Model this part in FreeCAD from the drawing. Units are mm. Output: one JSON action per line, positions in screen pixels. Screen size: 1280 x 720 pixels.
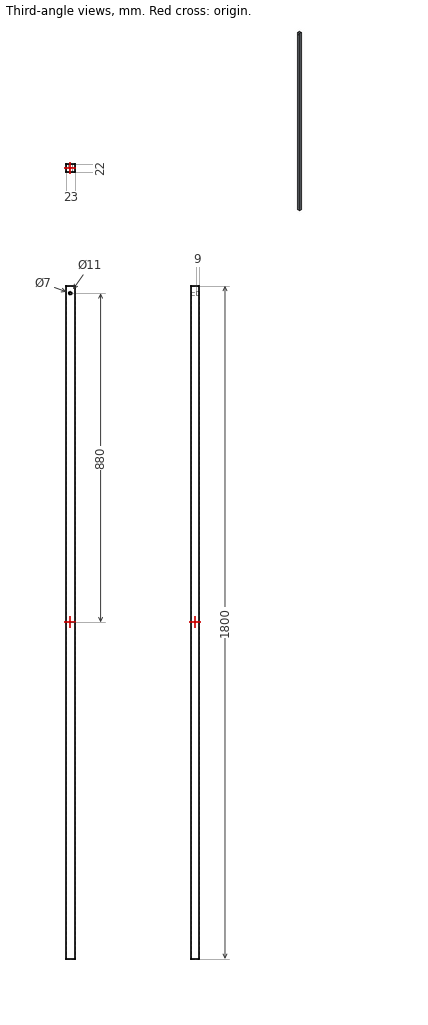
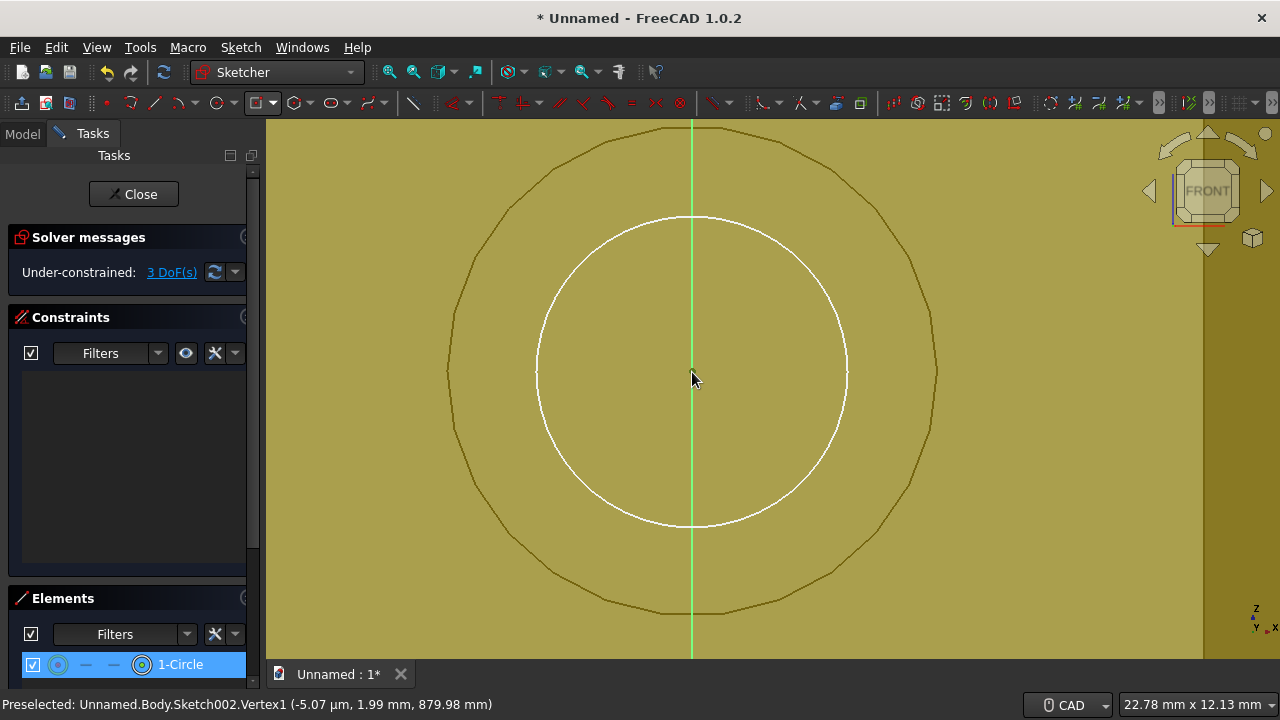
{"action": "left_click", "coordinate": [692, 596]}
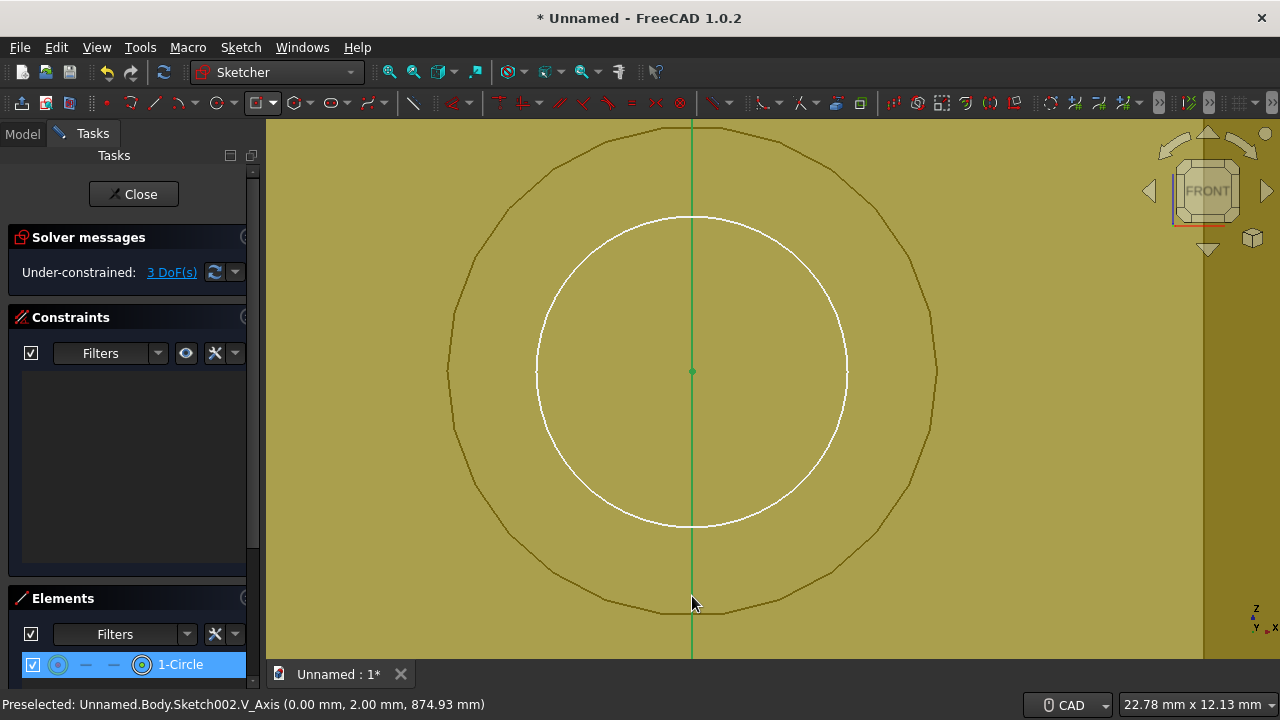
{"action": "left_click", "coordinate": [500, 104]}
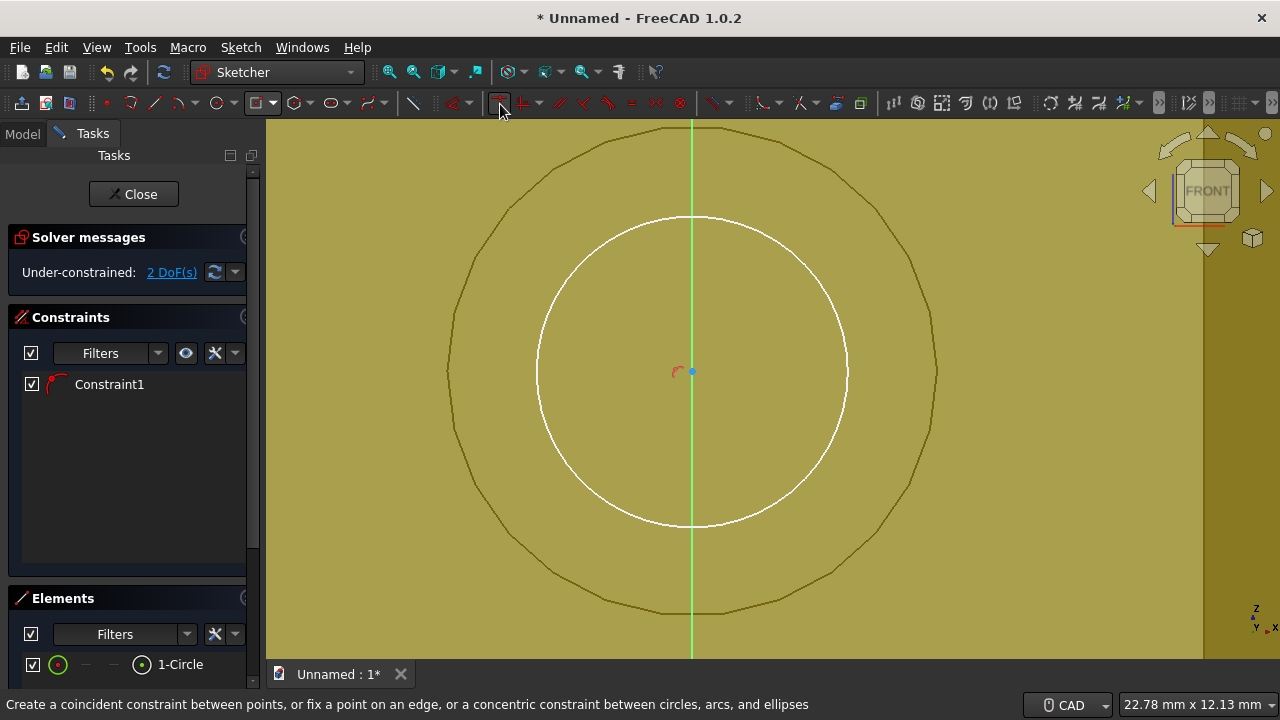
{"action": "left_click", "coordinate": [452, 104]}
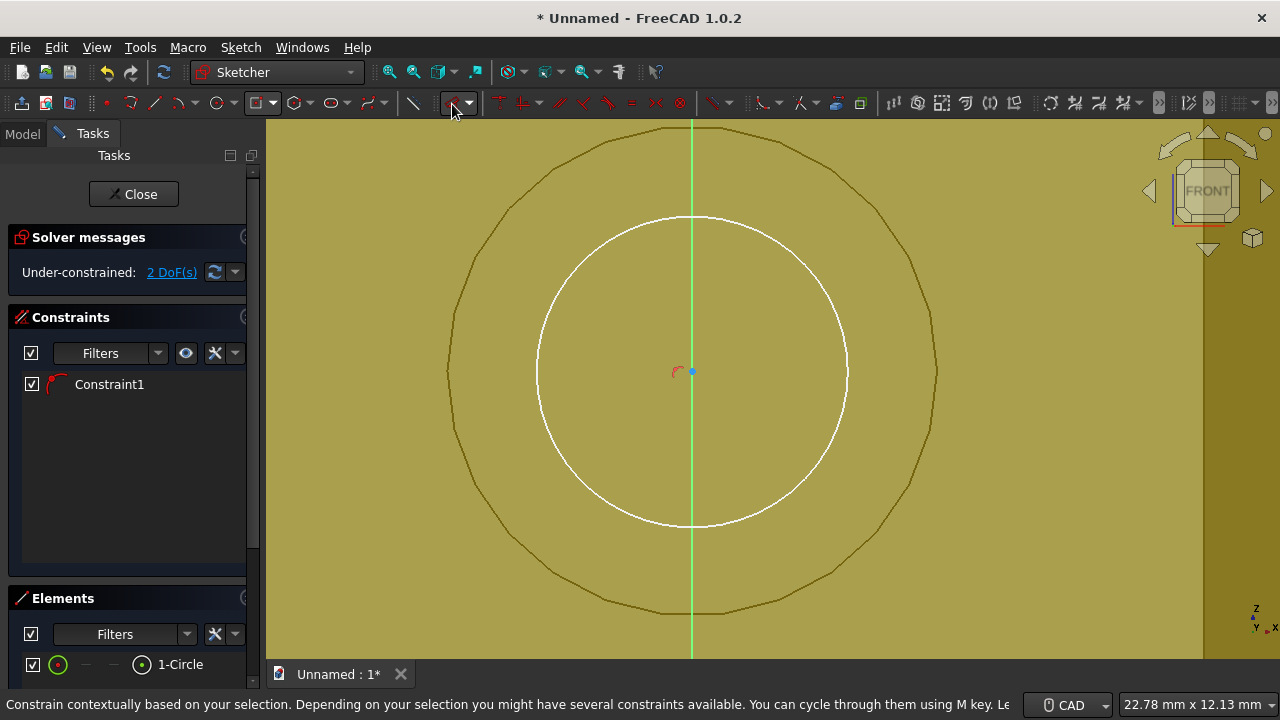
{"action": "left_click", "coordinate": [802, 262]}
{"action": "left_click", "coordinate": [825, 239]}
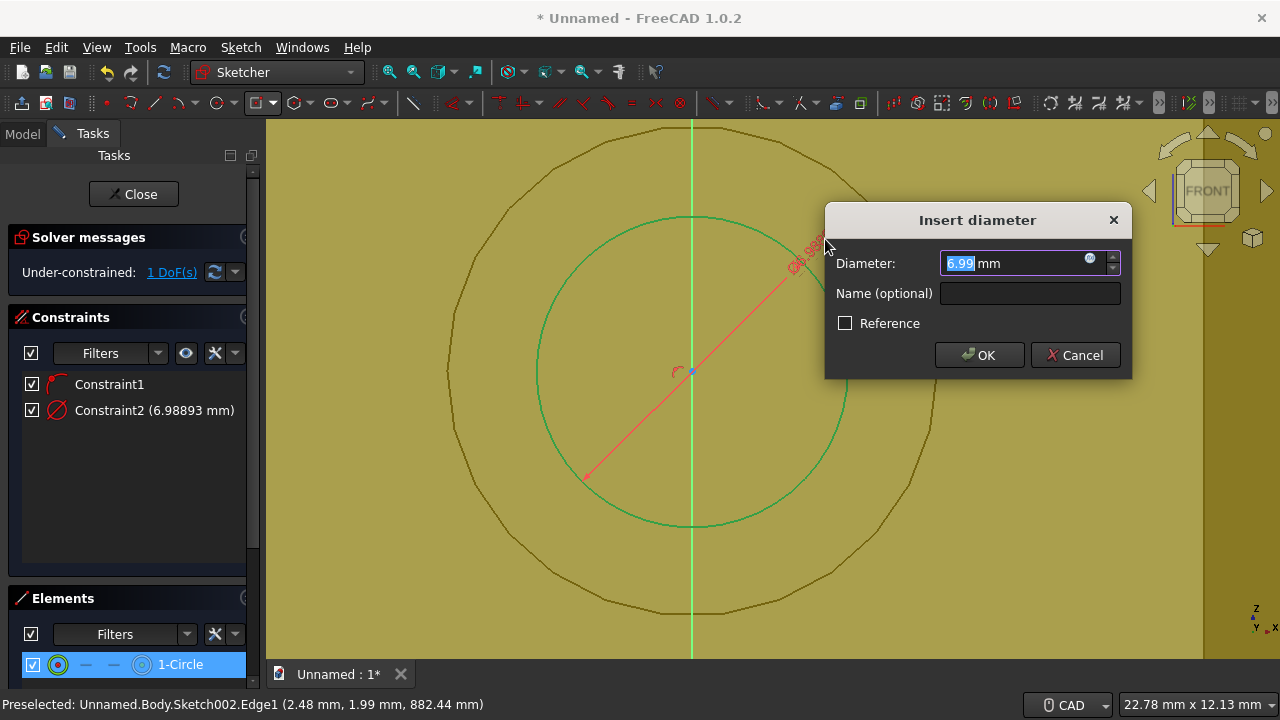
{"action": "type", "text": "7"}
{"action": "key", "text": "Return"}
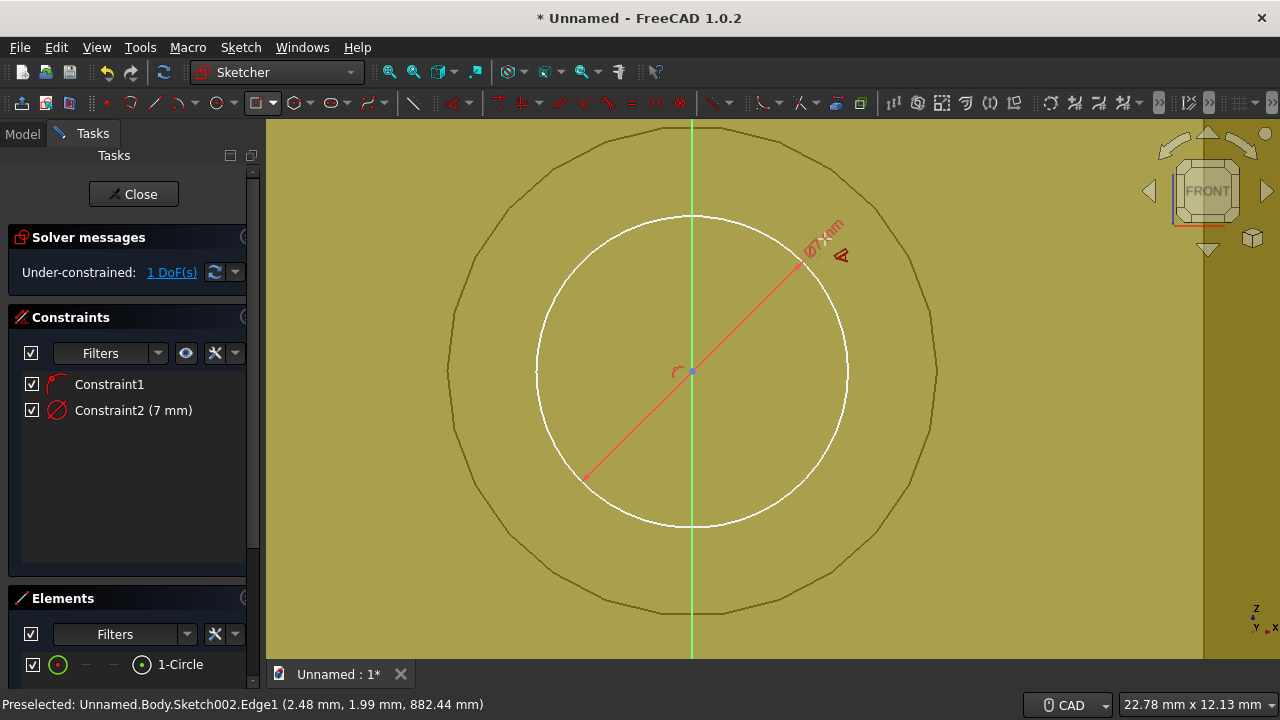
{"action": "left_click", "coordinate": [692, 372]}
{"action": "left_click", "coordinate": [726, 501]}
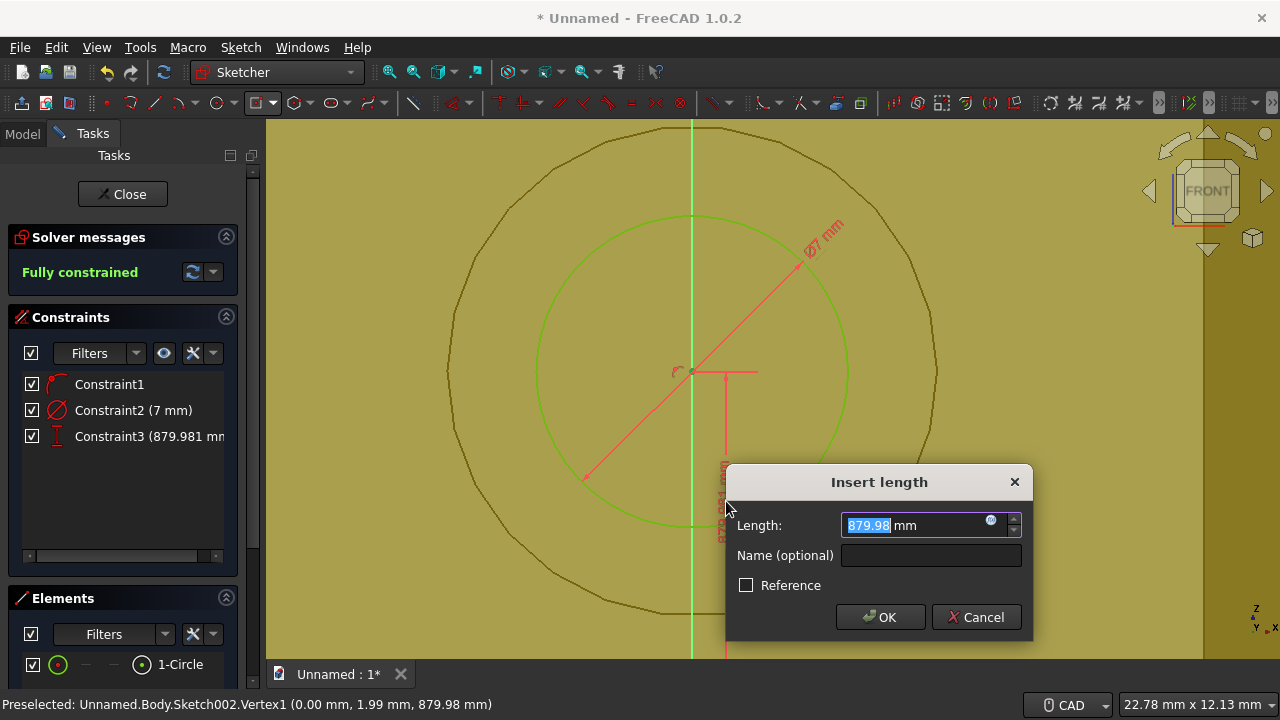
{"action": "type", "text": "880"}
{"action": "key", "text": "Return"}
{"action": "key", "text": "Escape"}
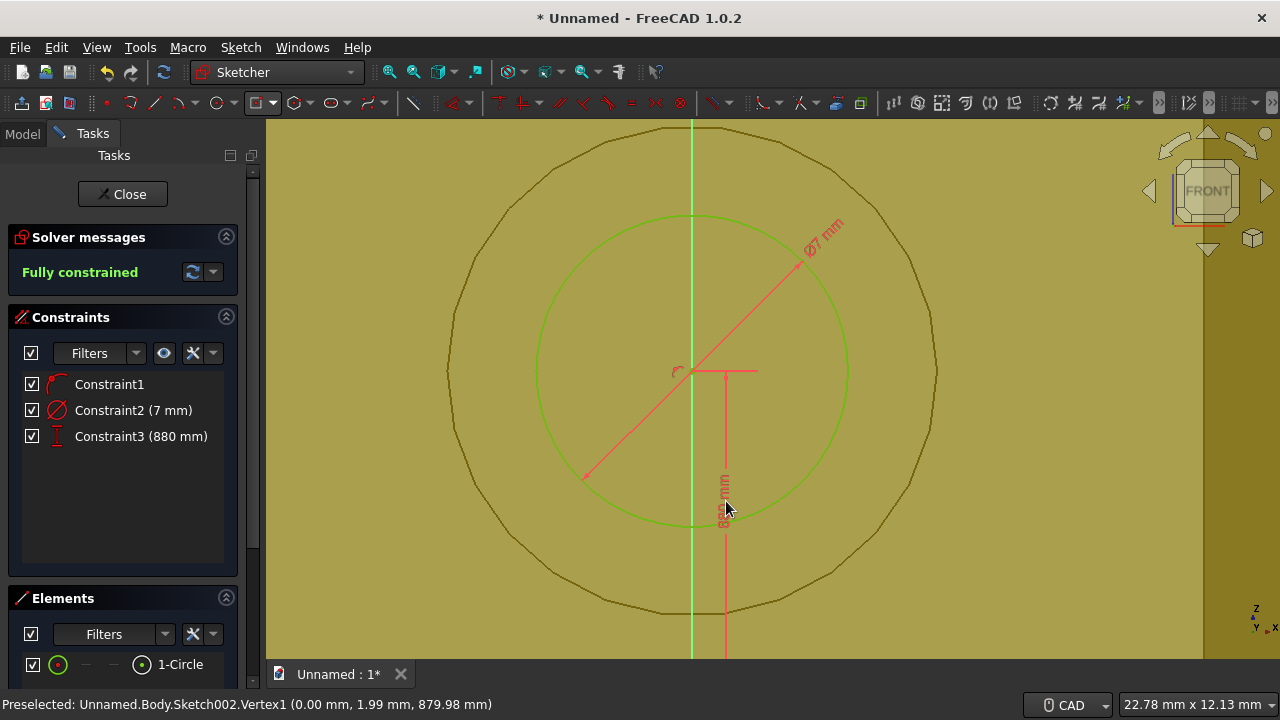
{"action": "left_click", "coordinate": [123, 194]}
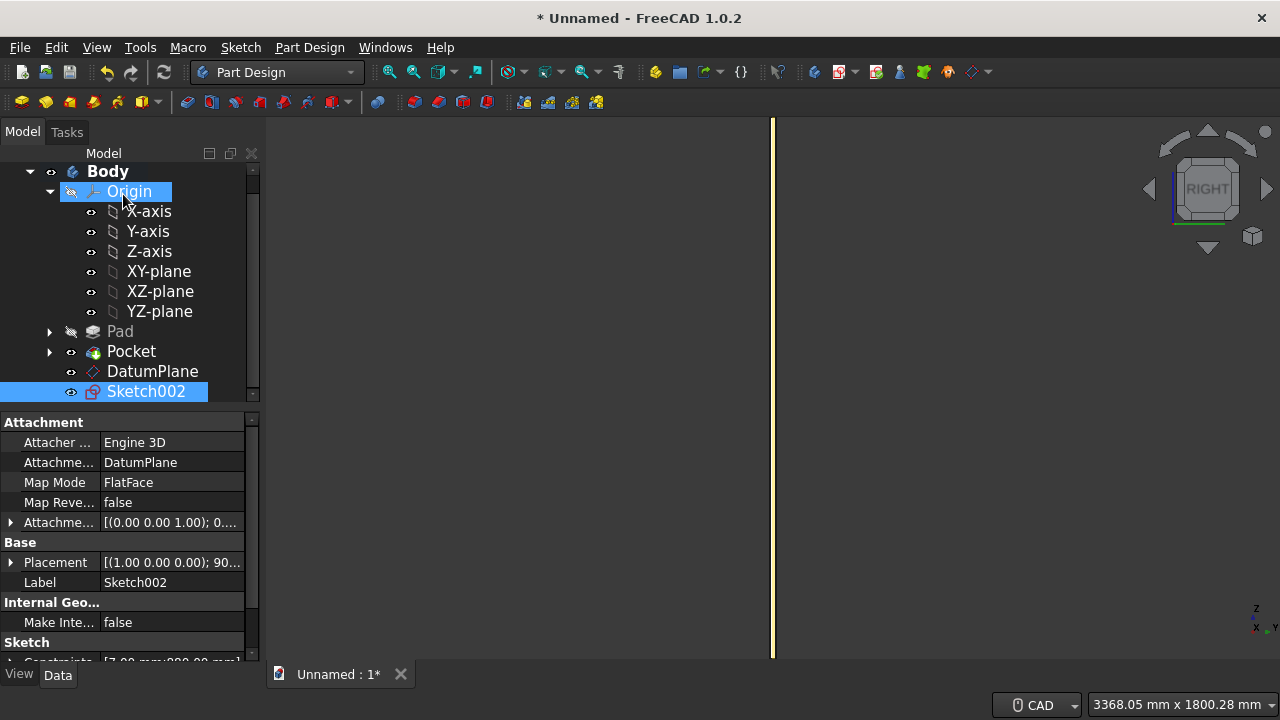
{"action": "left_click", "coordinate": [188, 102]}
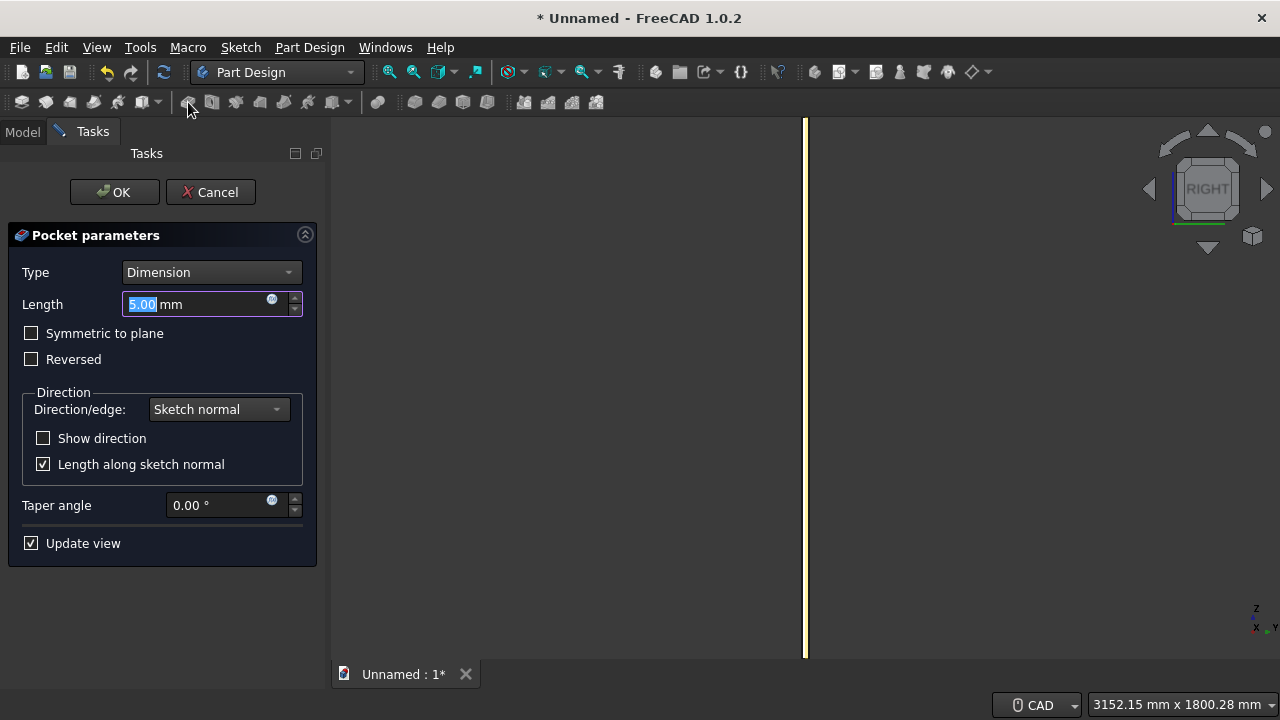
{"action": "left_click", "coordinate": [212, 272]}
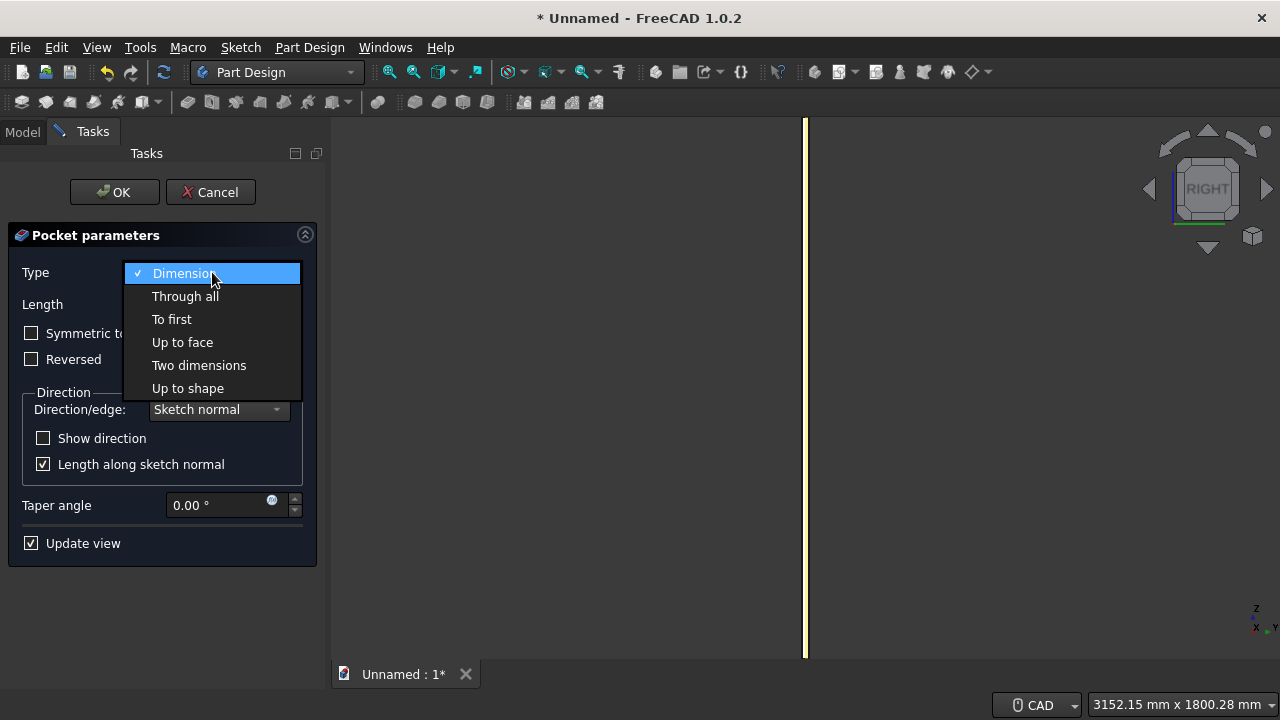
{"action": "left_click", "coordinate": [212, 320]}